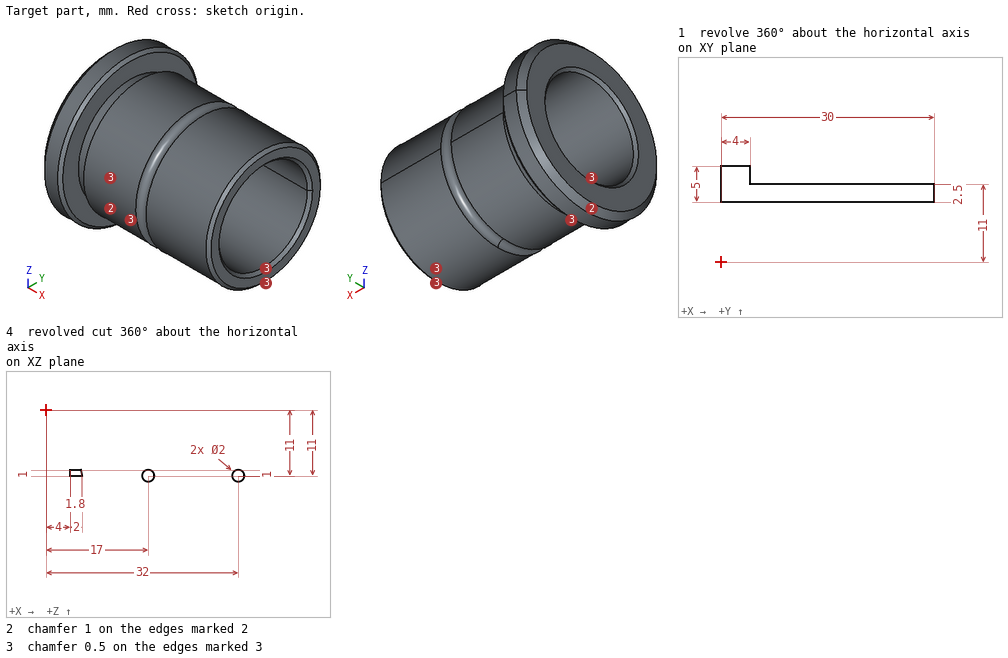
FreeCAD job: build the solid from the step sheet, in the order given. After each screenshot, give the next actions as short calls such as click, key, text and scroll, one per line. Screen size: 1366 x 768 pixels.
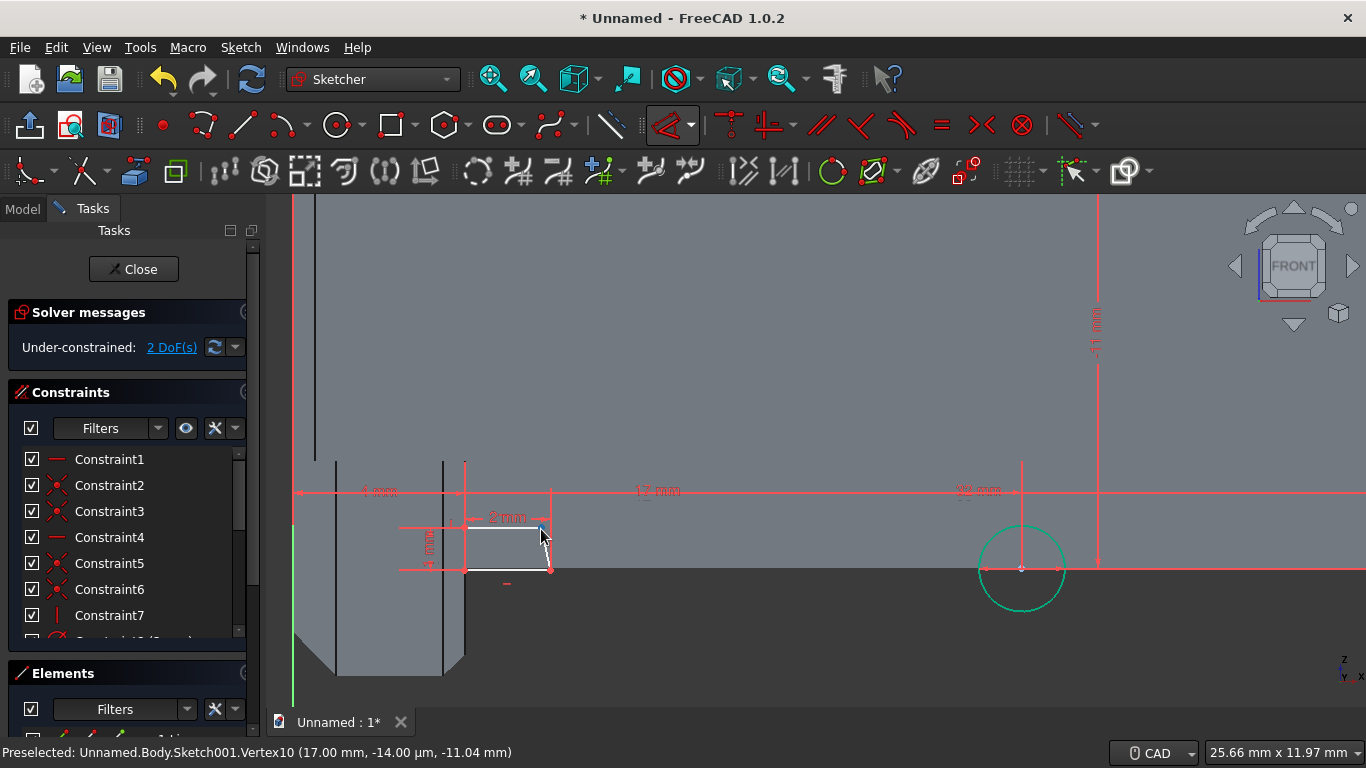
click(541, 528)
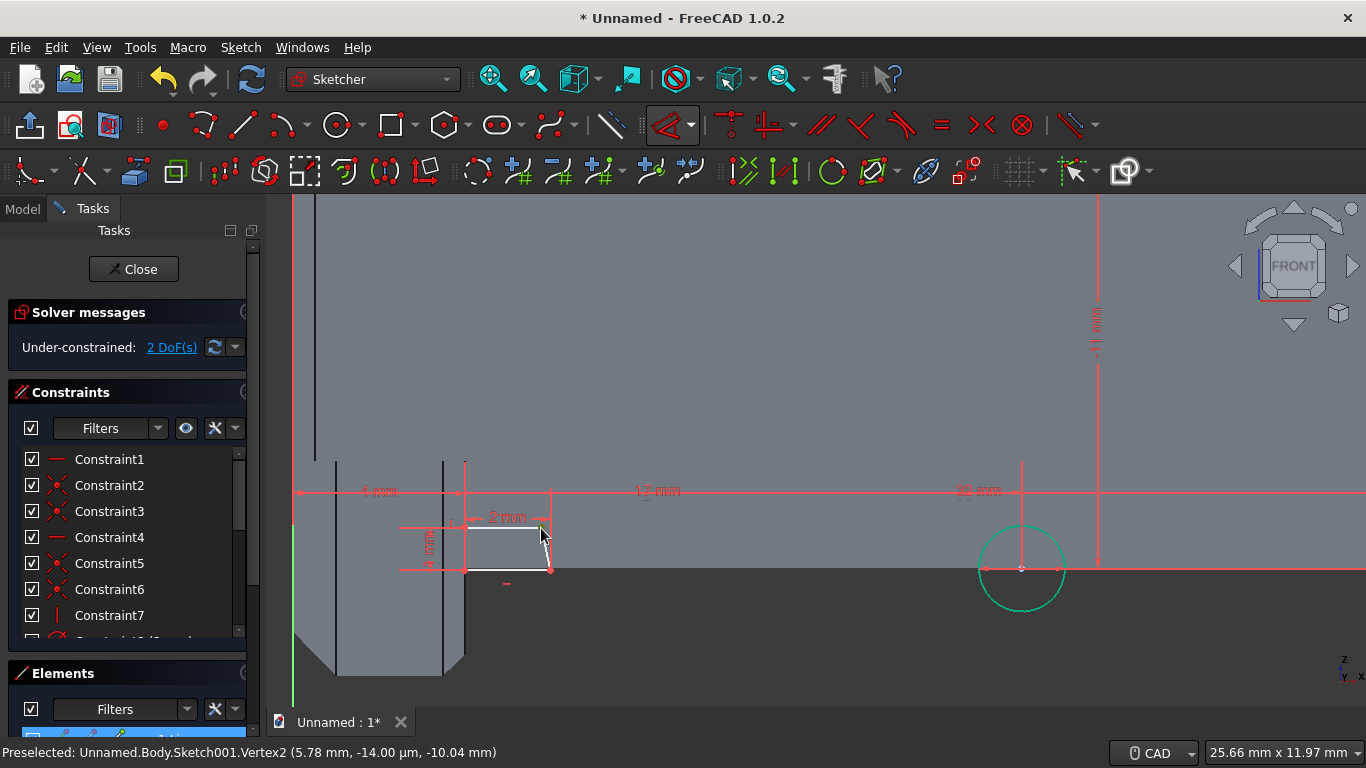
scroll(541, 529, down, 4)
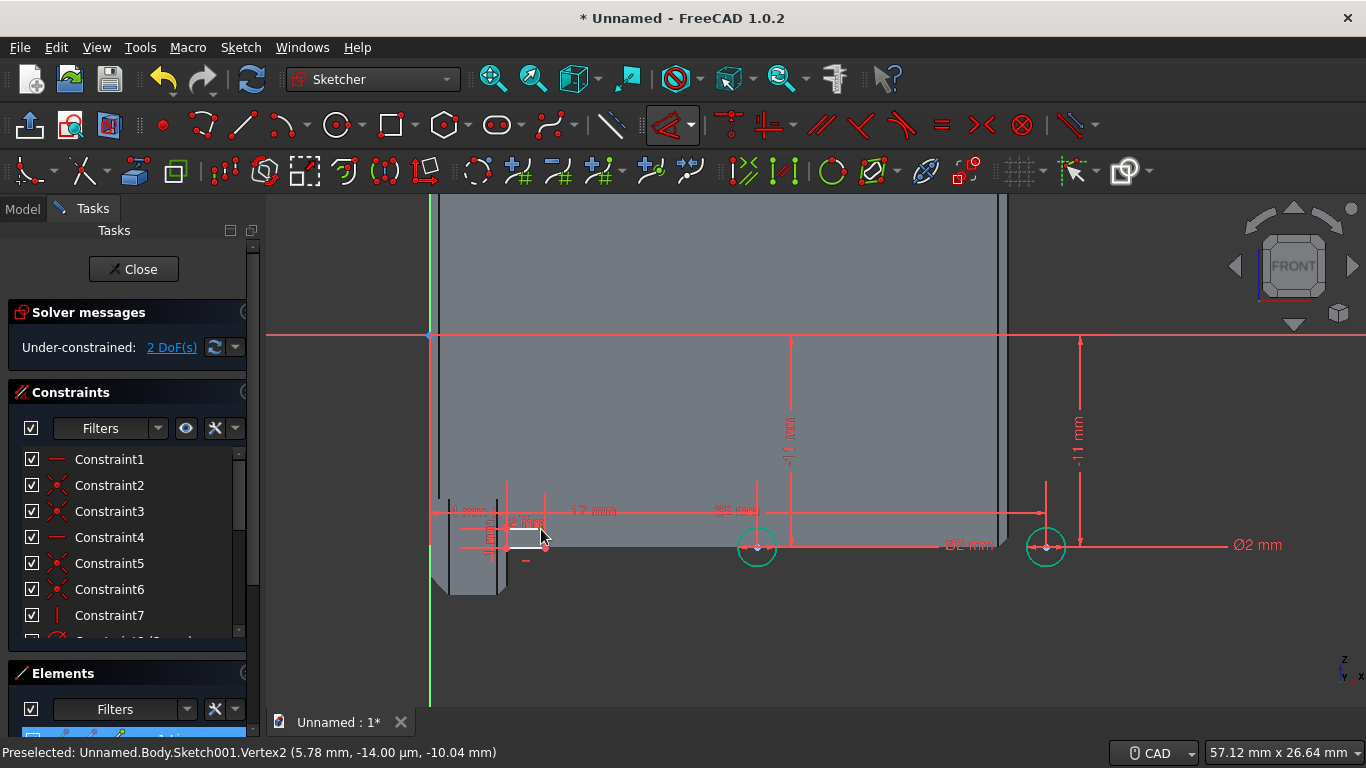
scroll(1046, 547, up, 4)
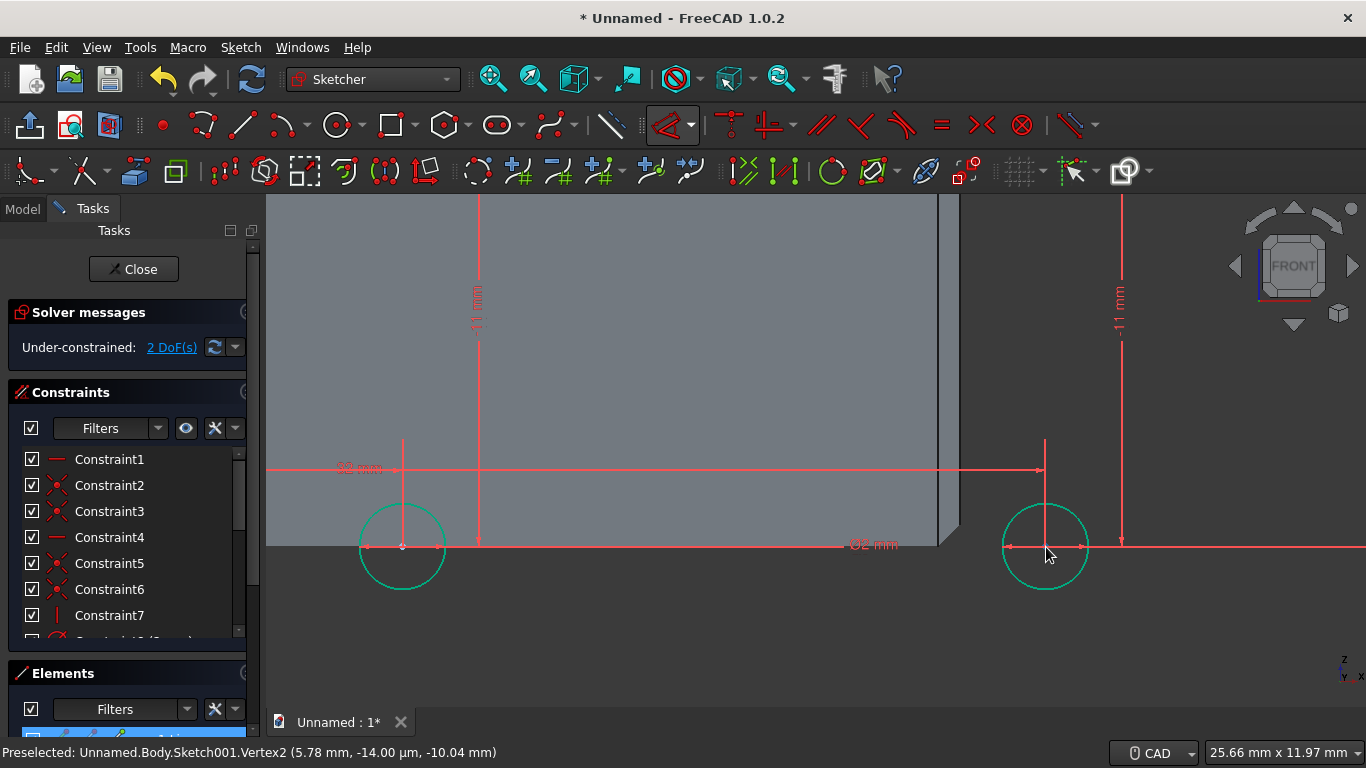
click(1045, 547)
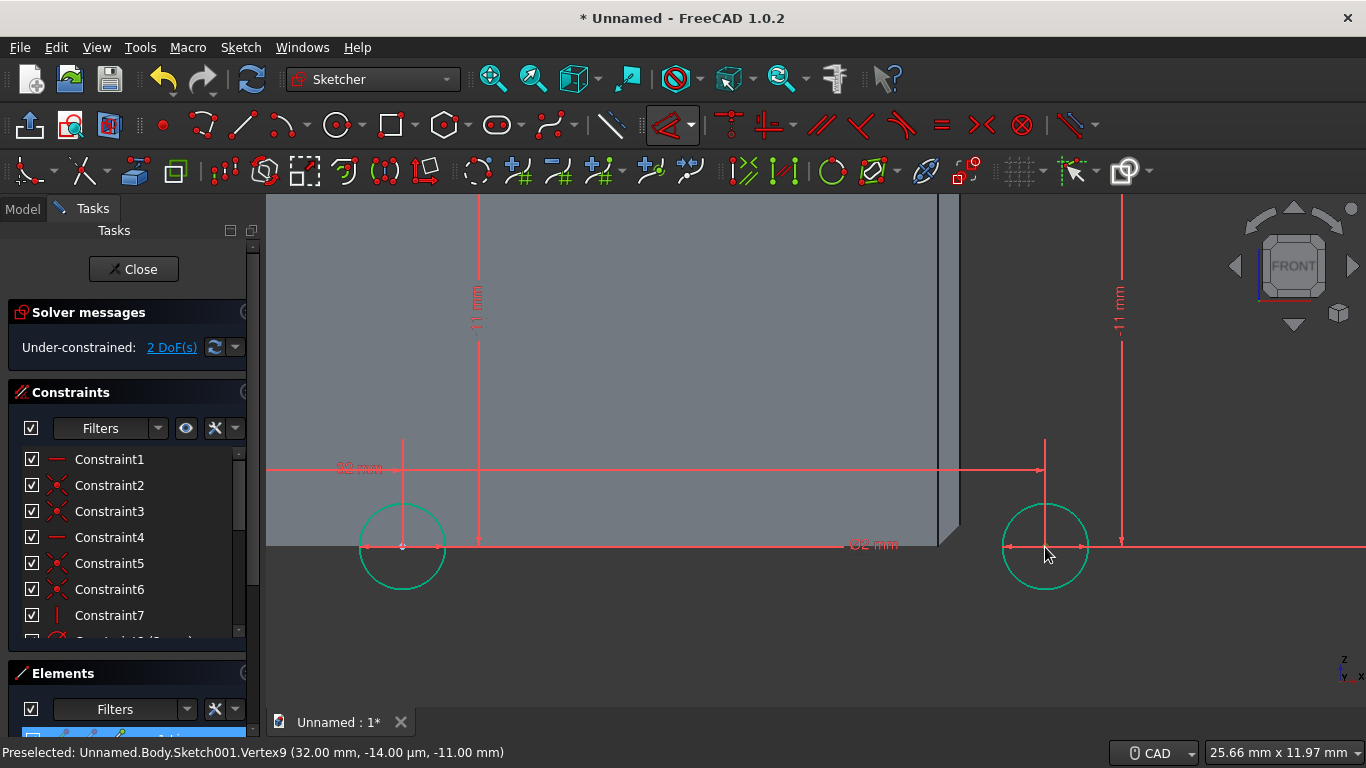
key(i)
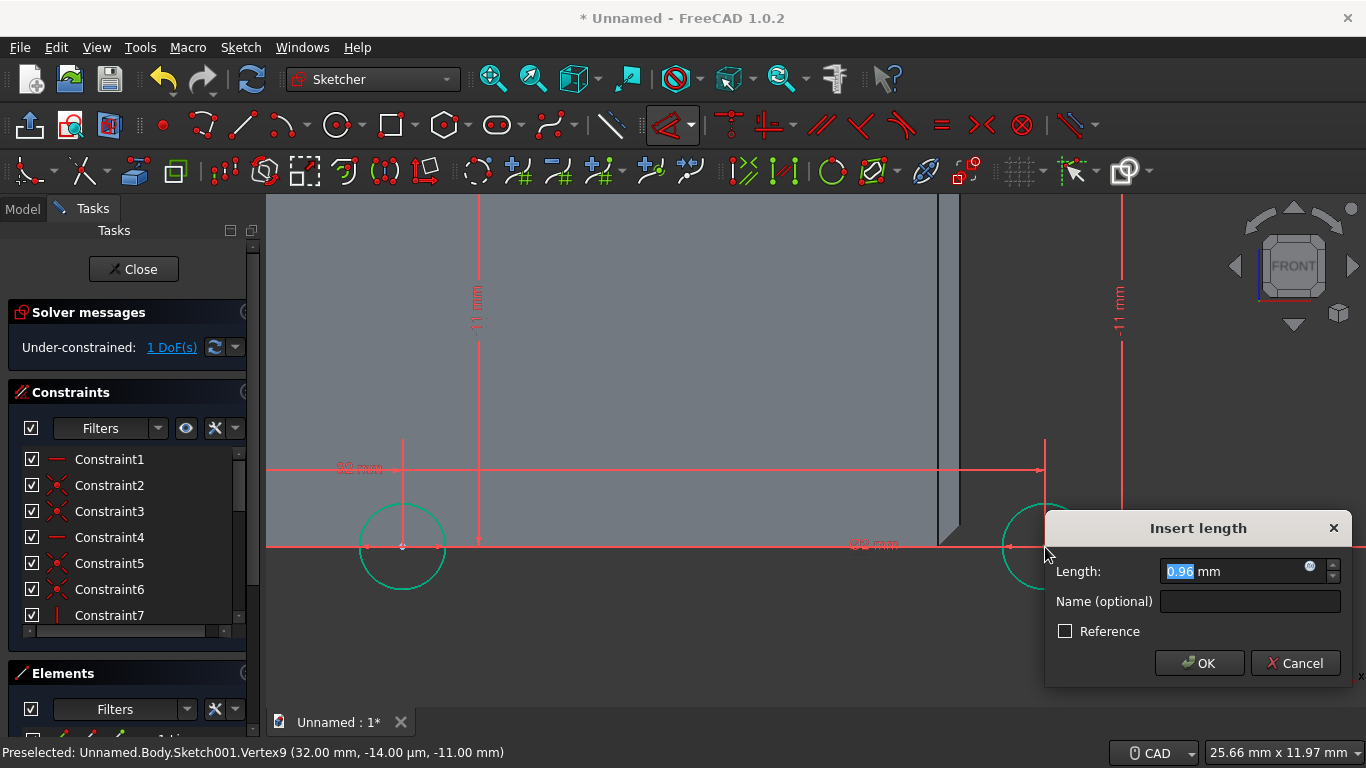
text(1)
key(Return)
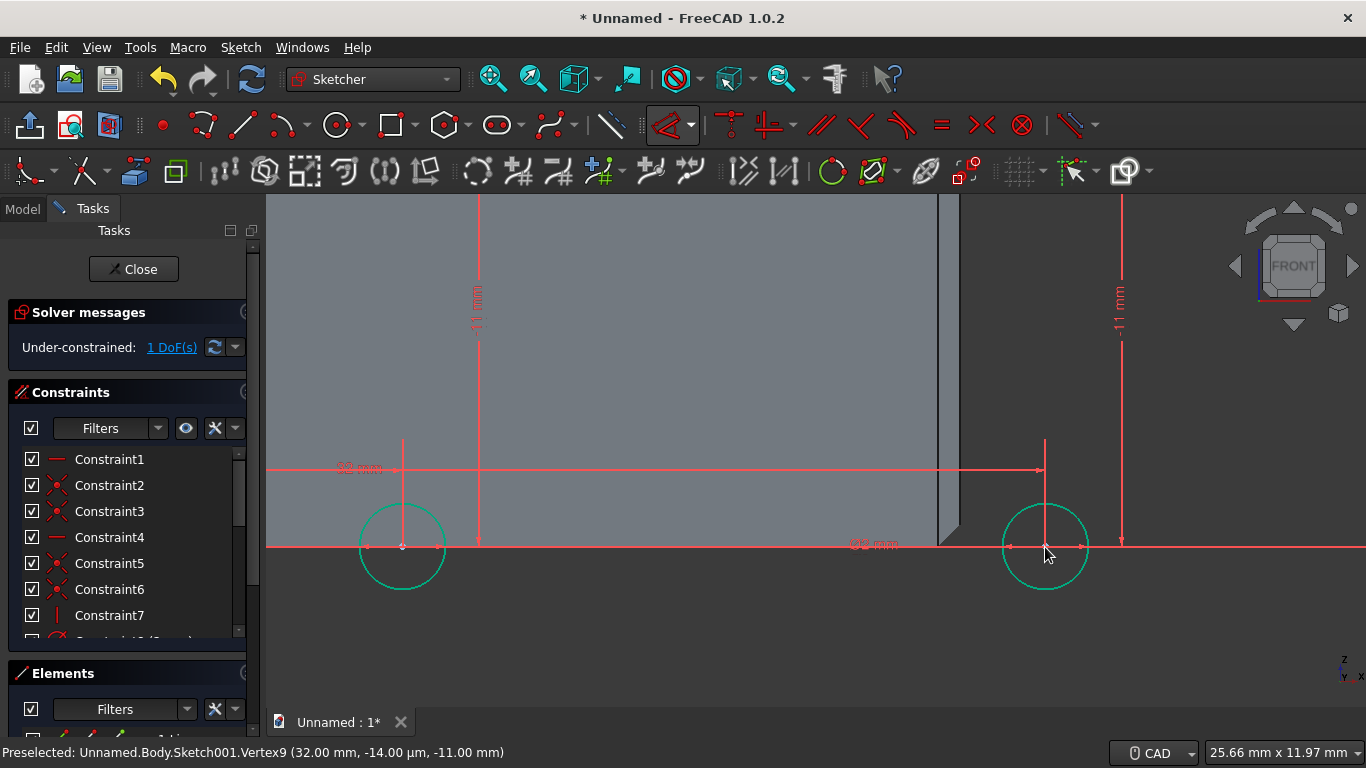
scroll(1046, 547, down, 4)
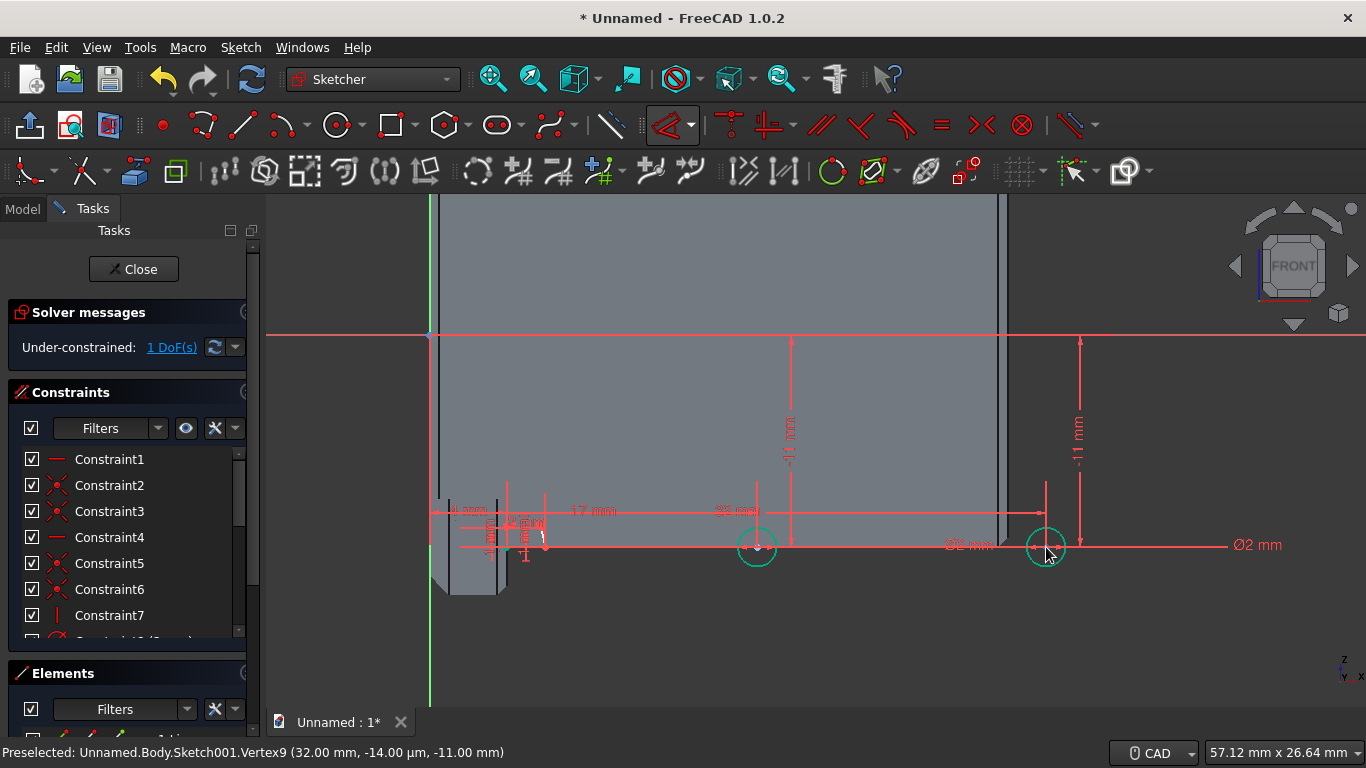
scroll(517, 528, up, 2)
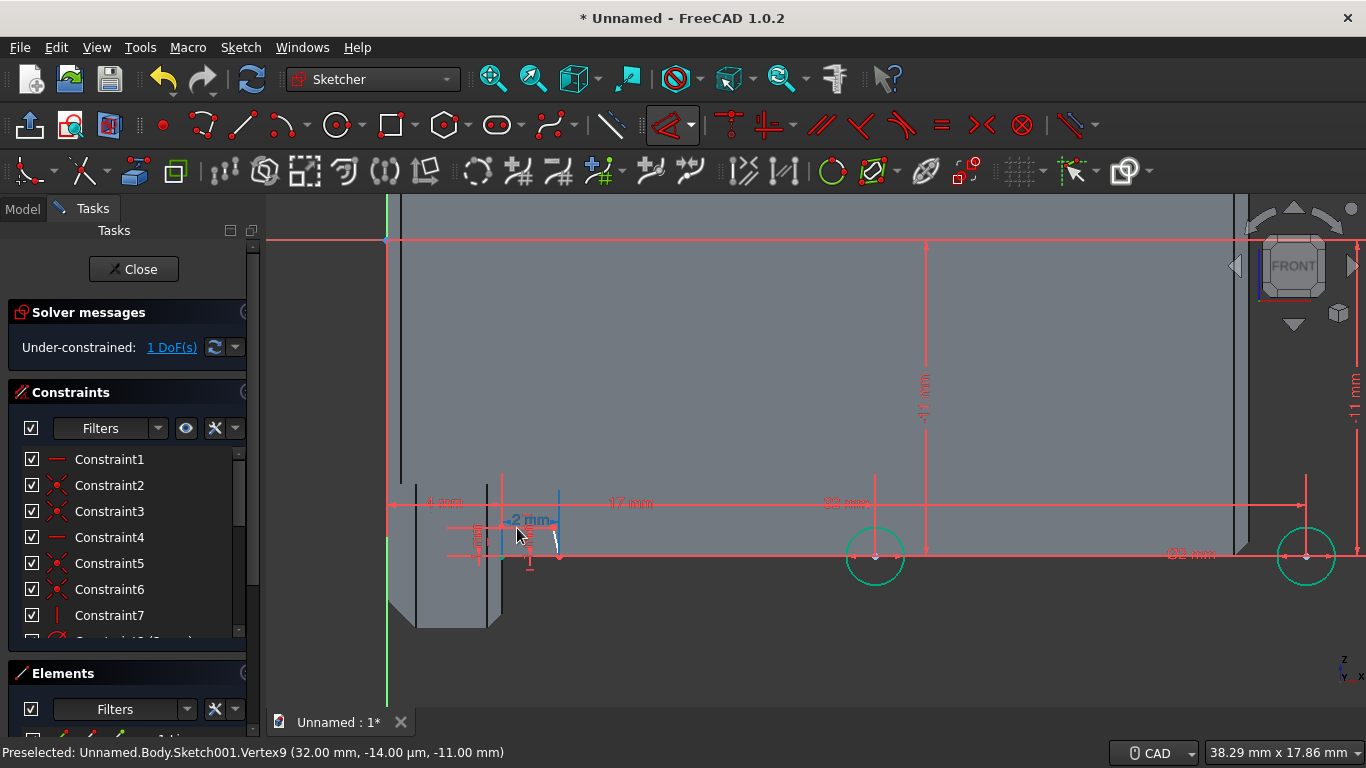
click(512, 528)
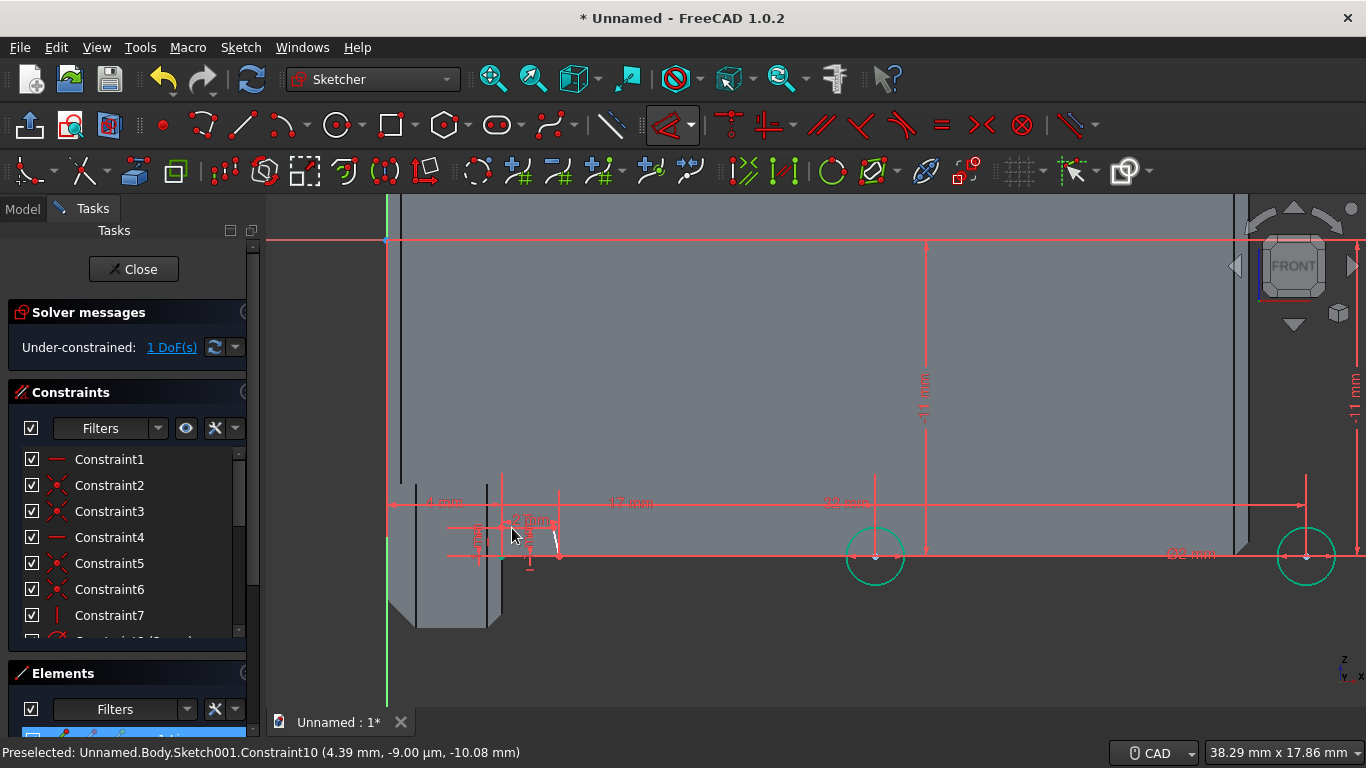
click(694, 126)